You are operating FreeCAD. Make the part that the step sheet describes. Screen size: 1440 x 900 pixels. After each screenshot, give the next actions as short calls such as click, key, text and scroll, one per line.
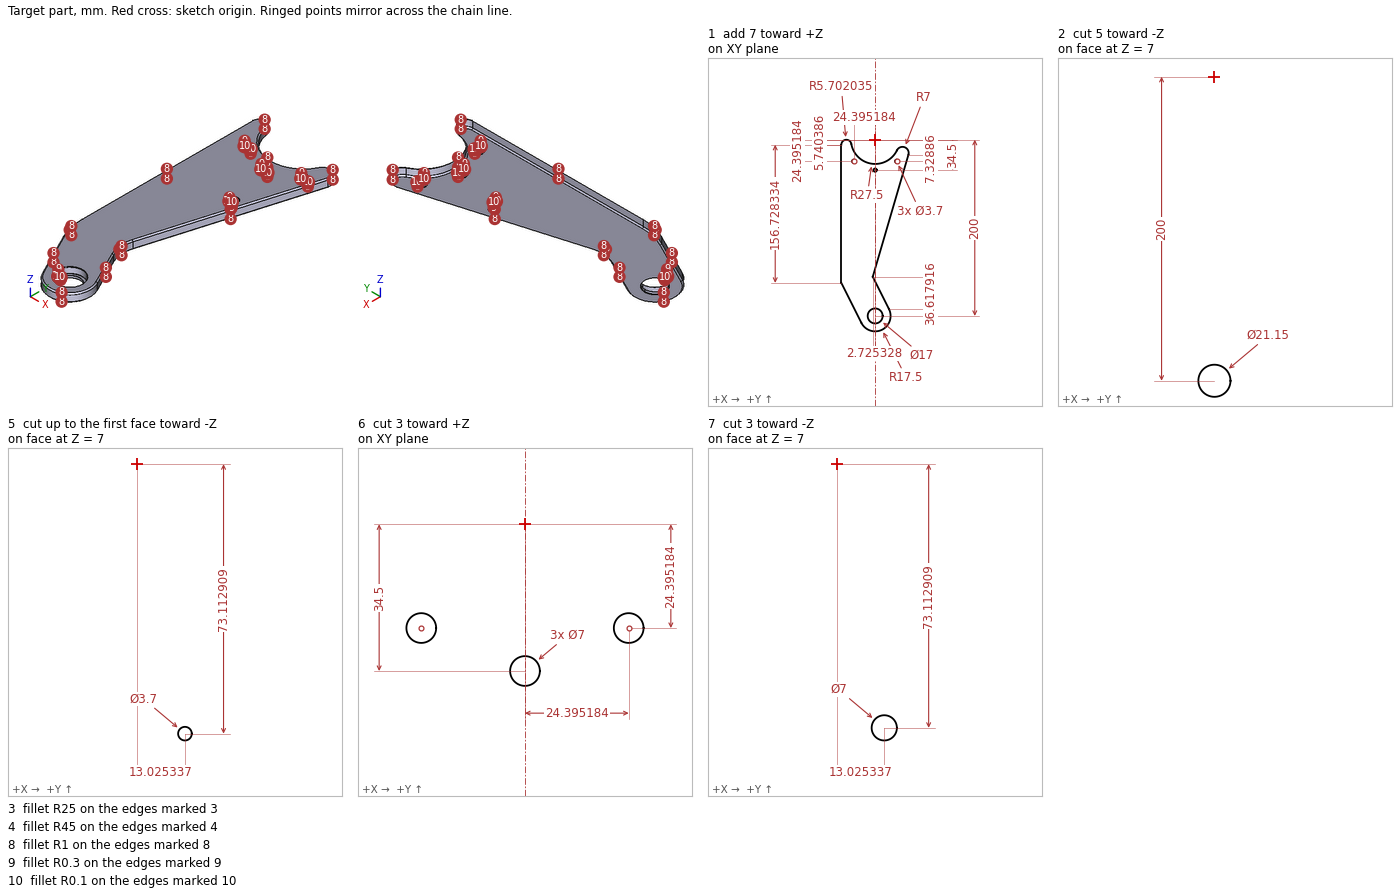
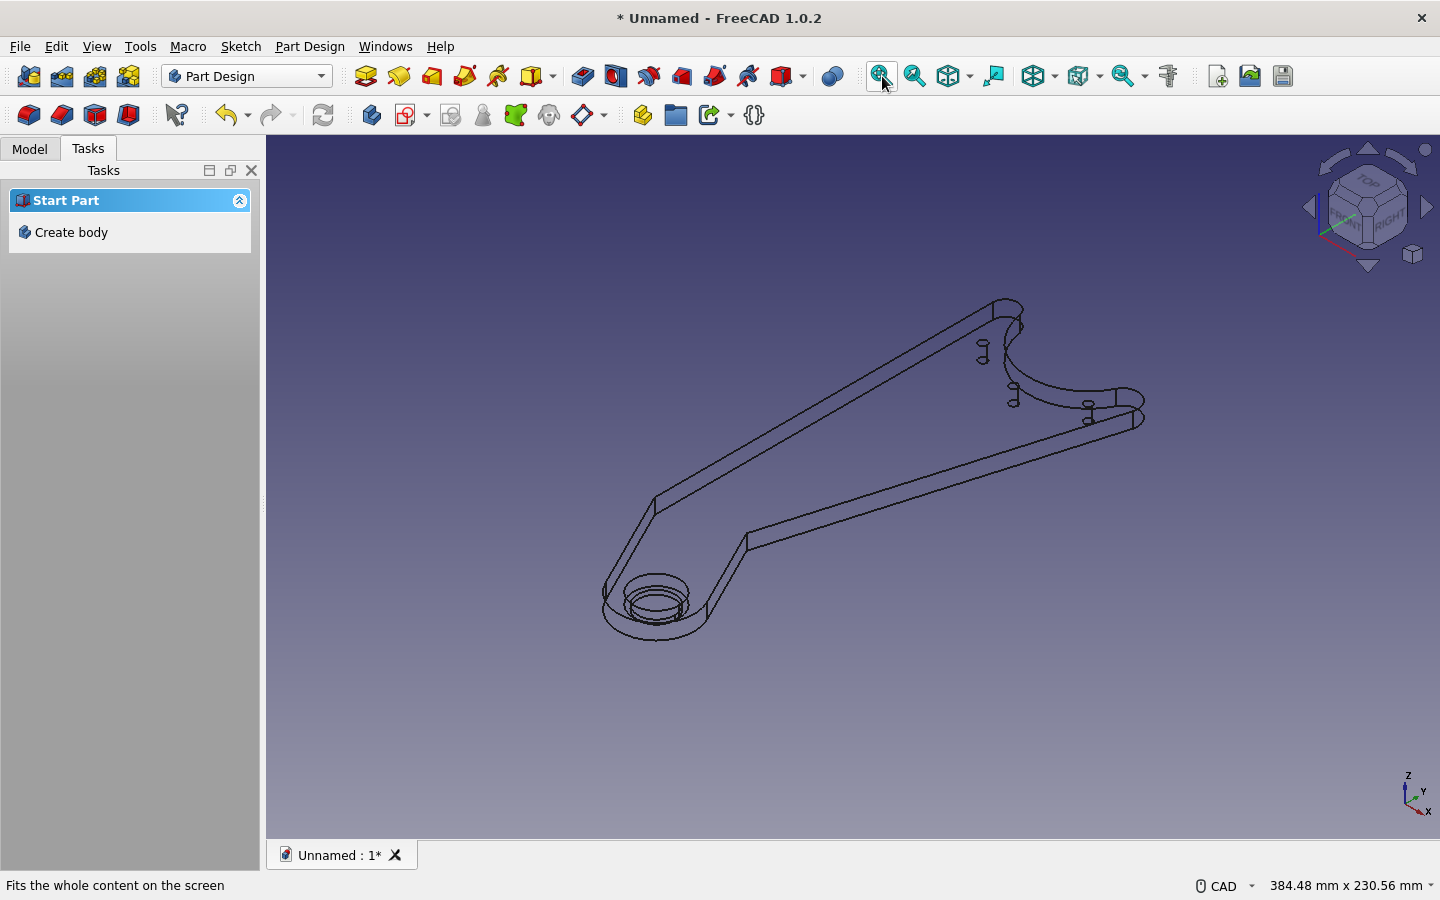
click(747, 545)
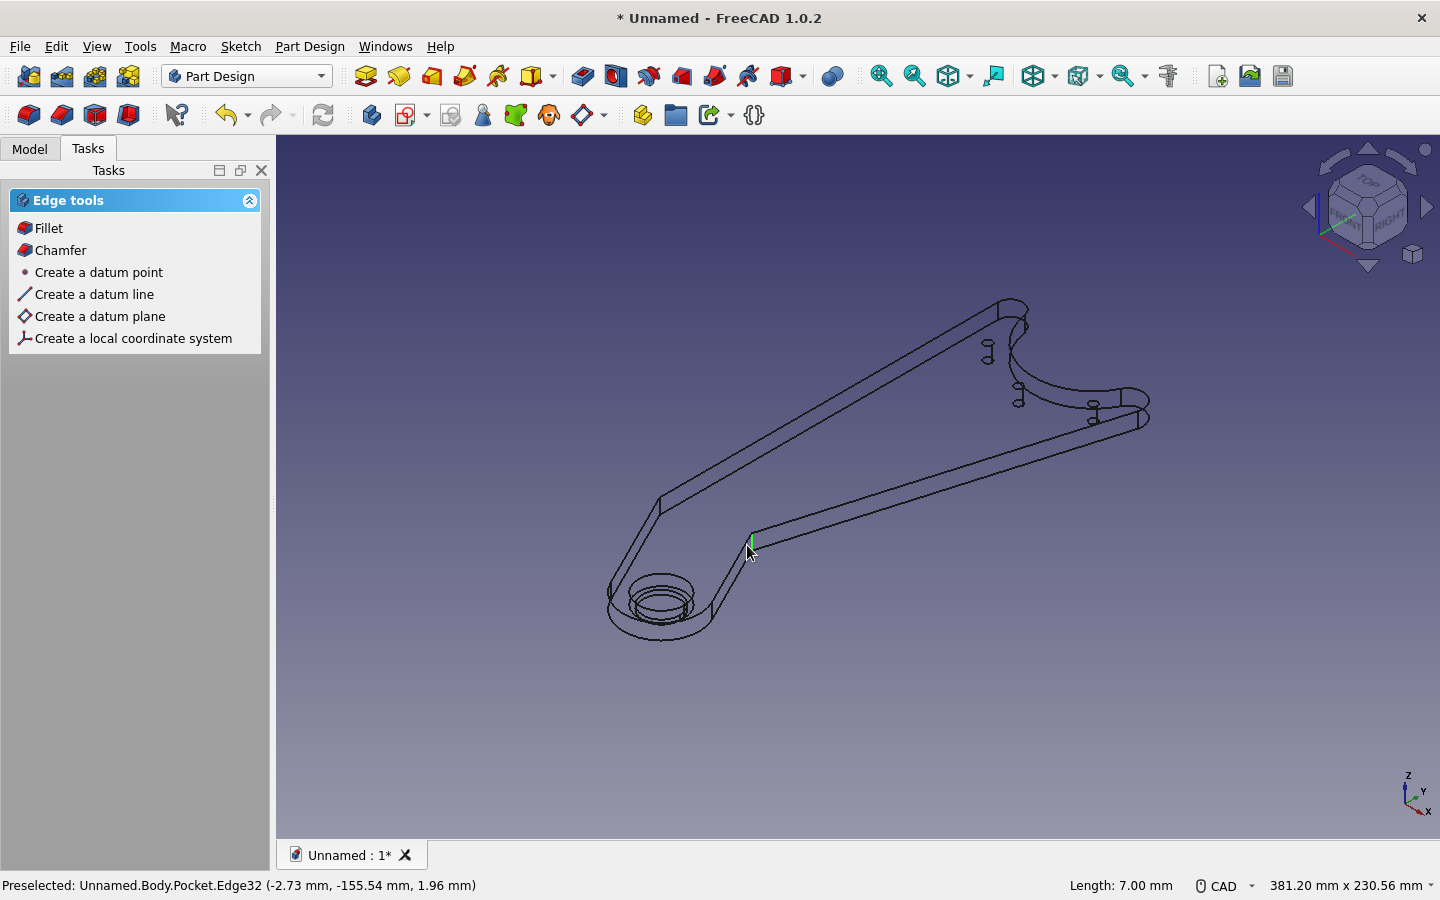
key(v)
key(1)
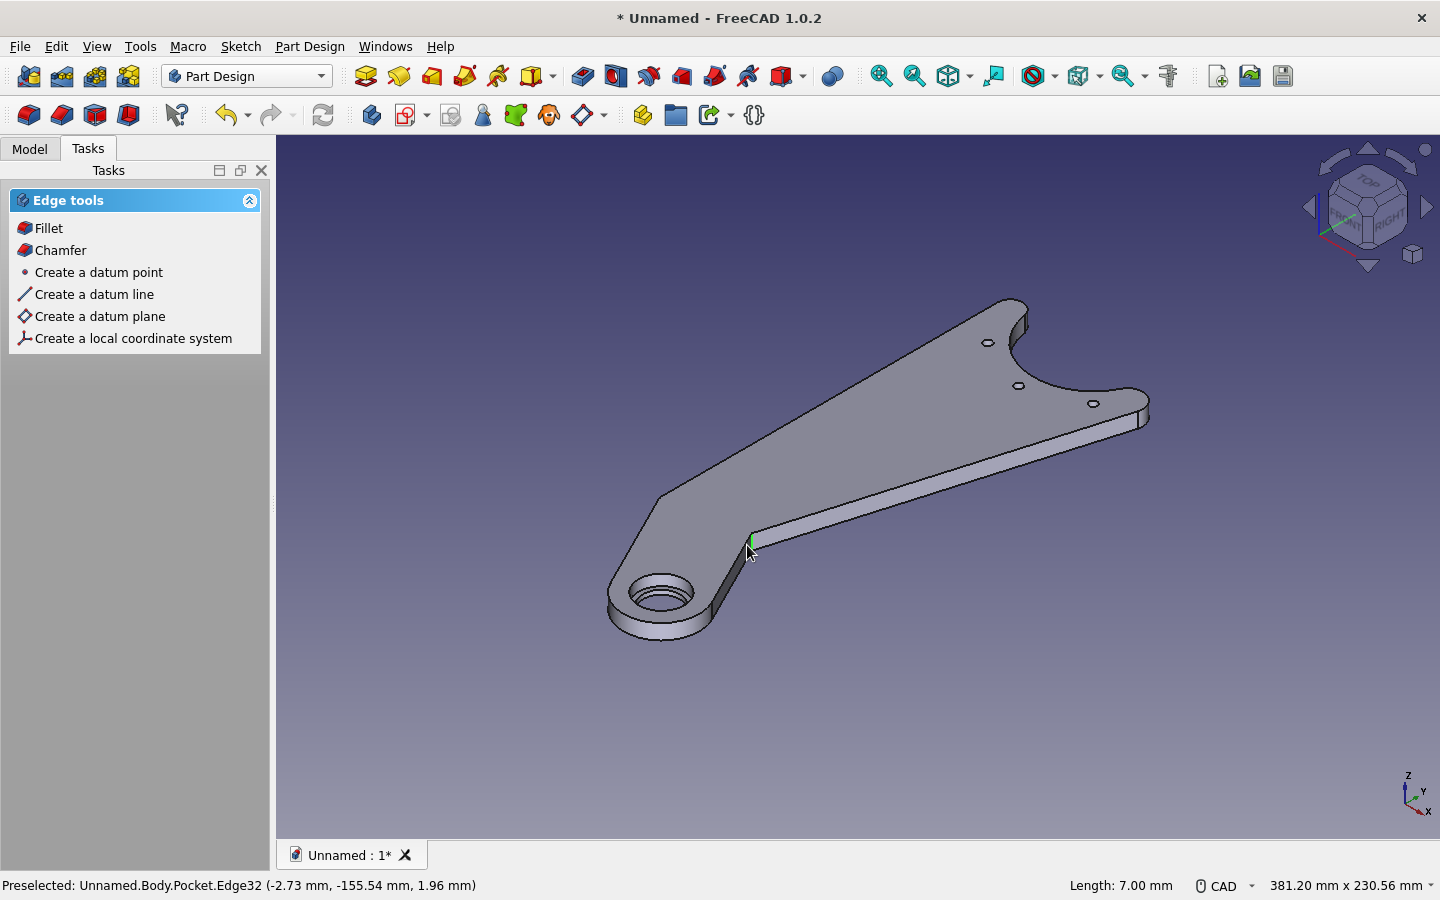
click(29, 116)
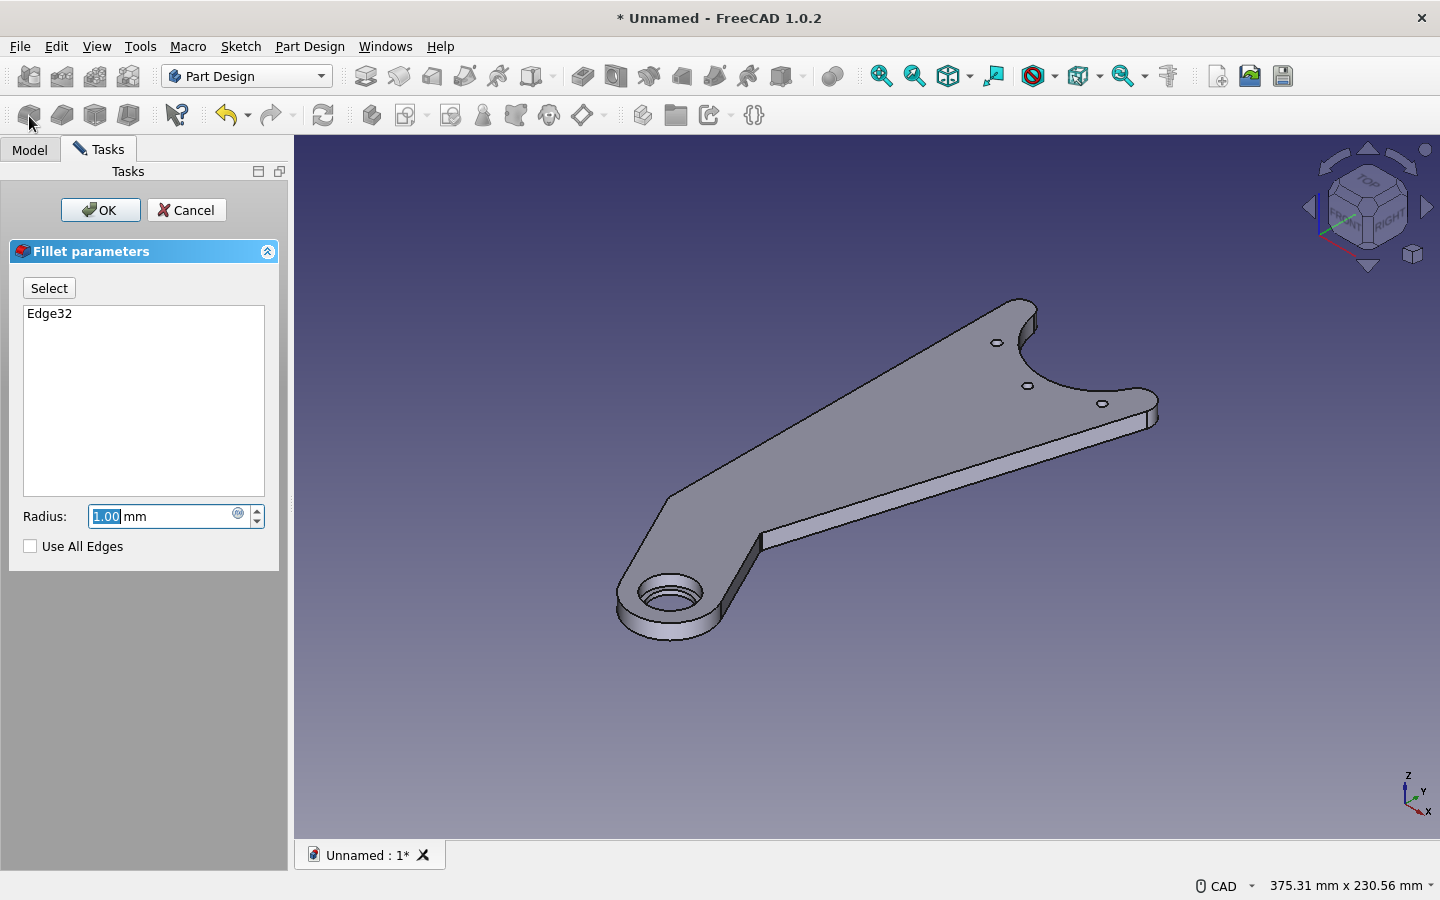
text(25)
key(Tab)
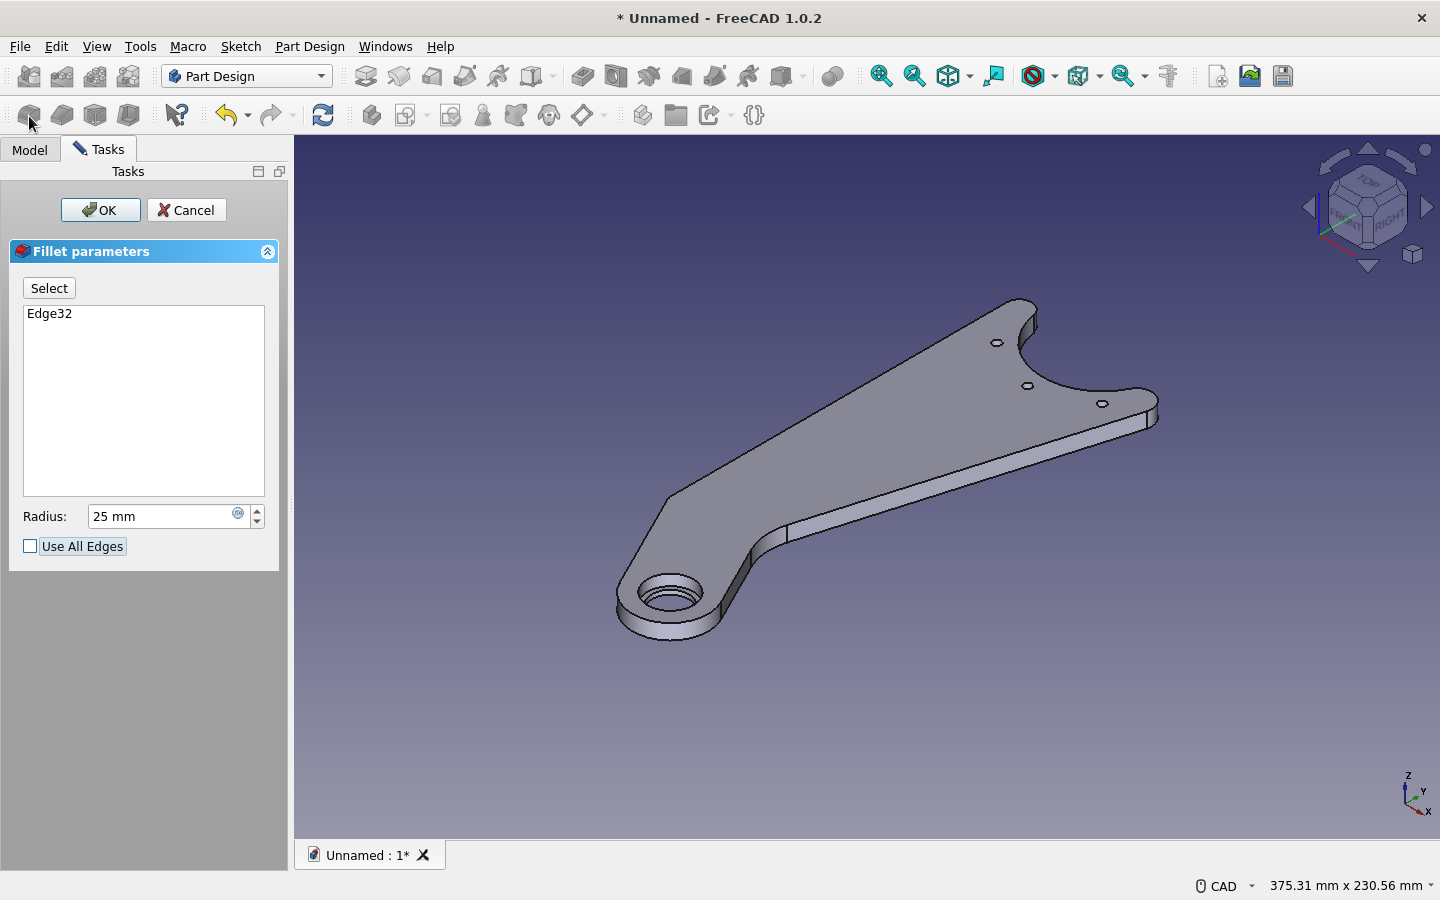
click(101, 210)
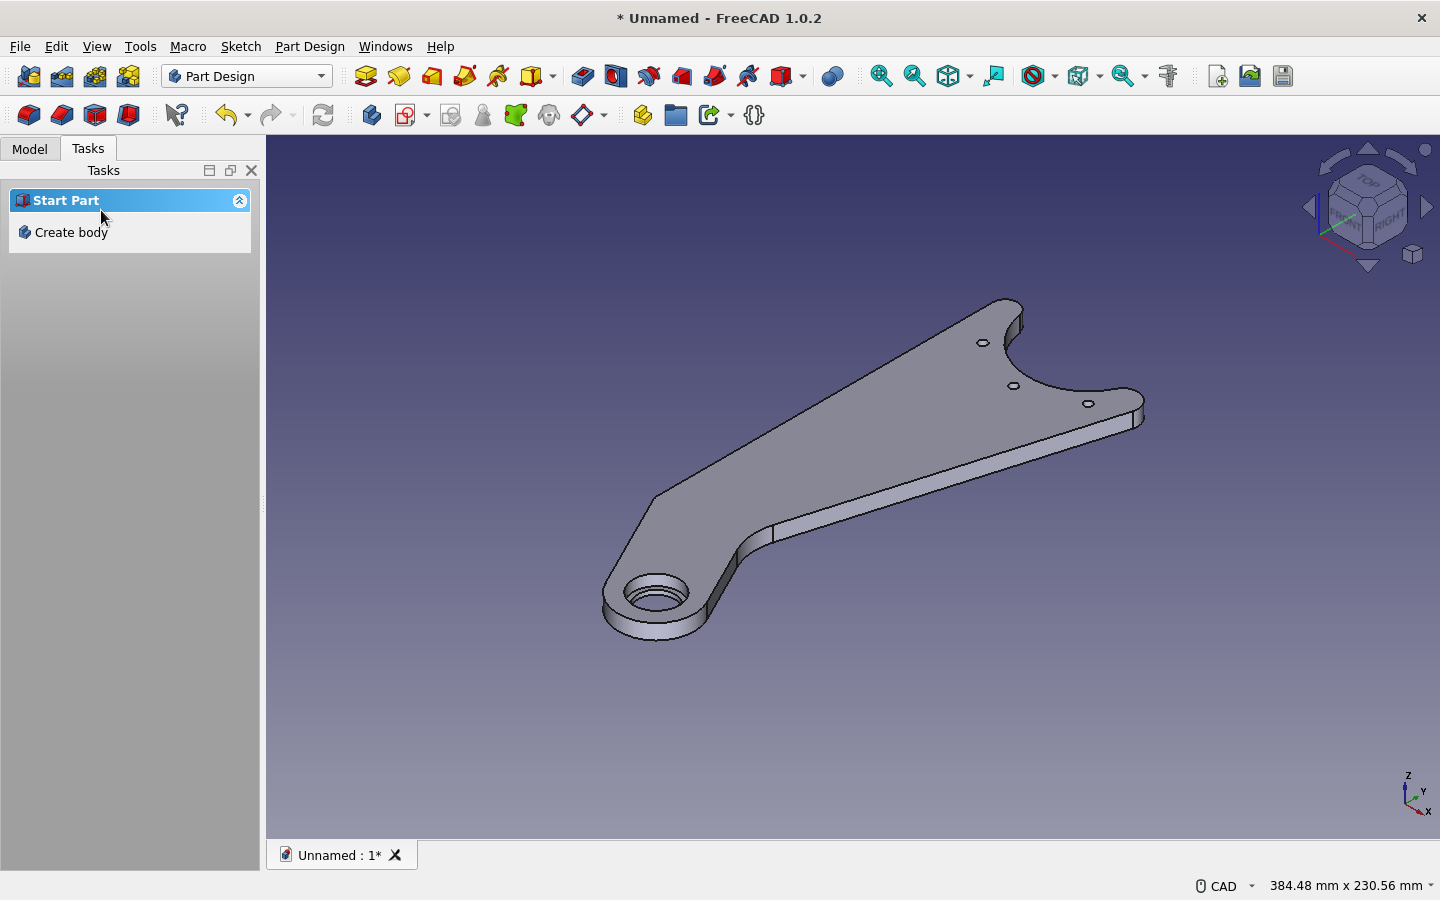
scroll(655, 505, up, 4)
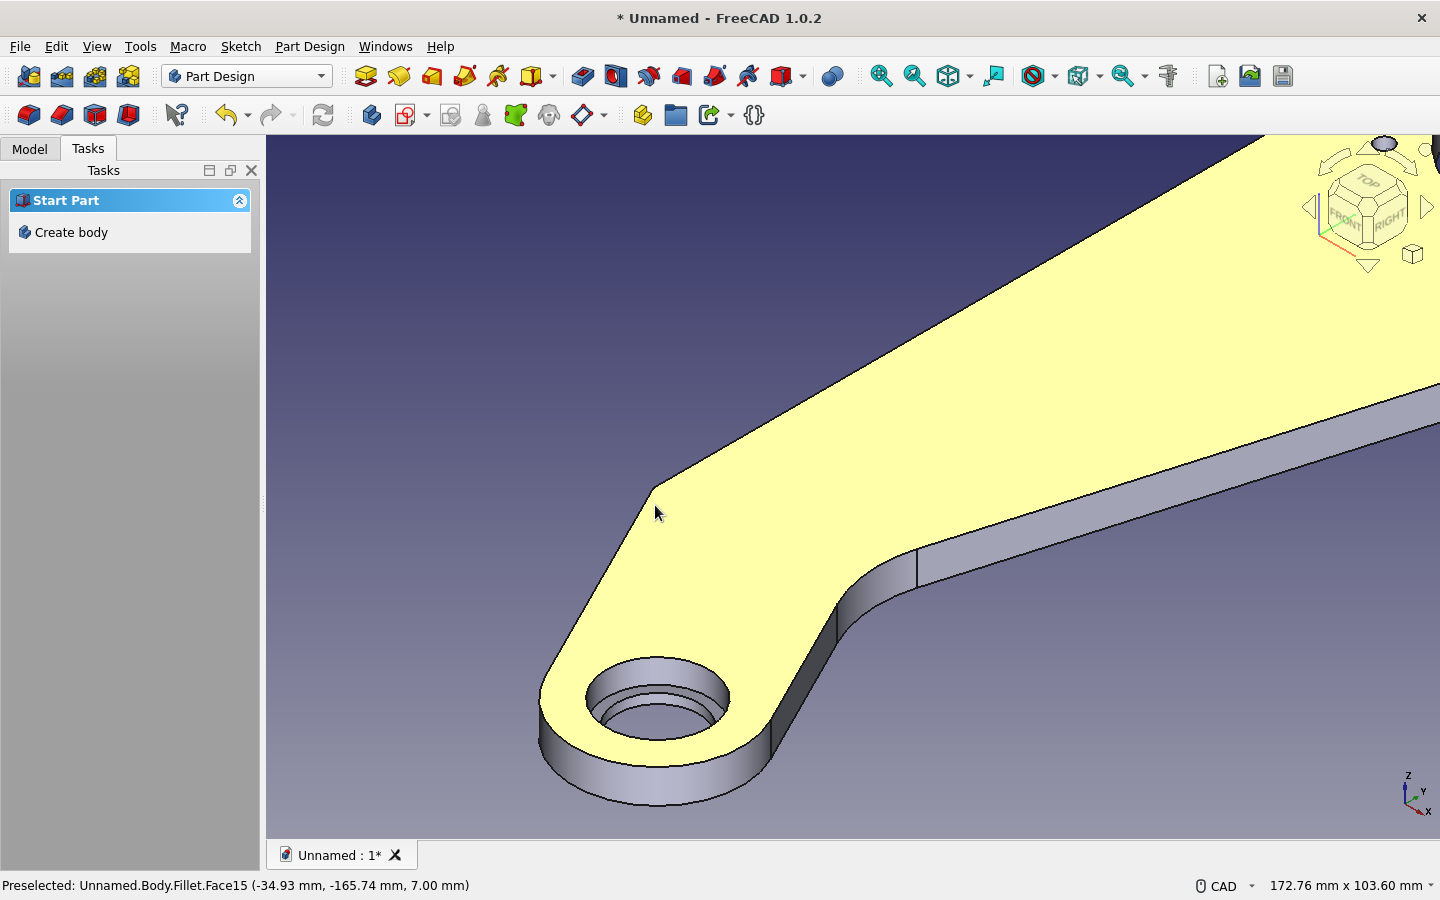
click(882, 76)